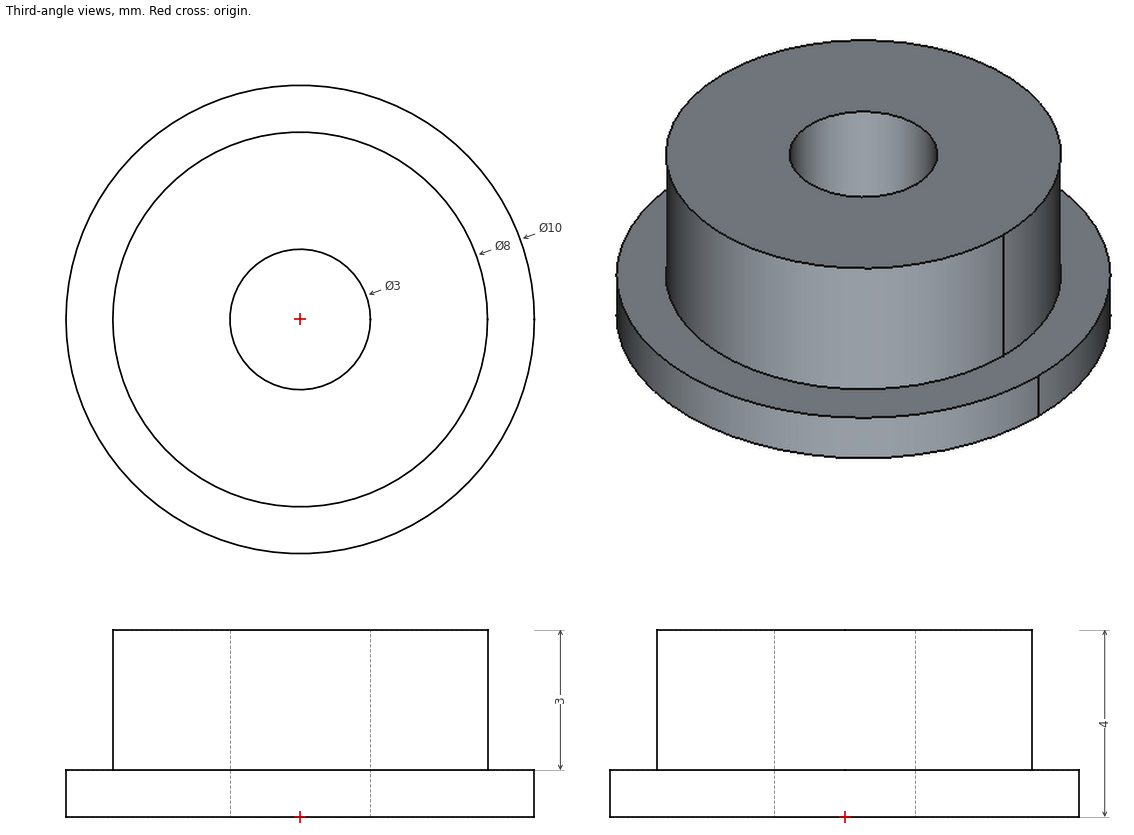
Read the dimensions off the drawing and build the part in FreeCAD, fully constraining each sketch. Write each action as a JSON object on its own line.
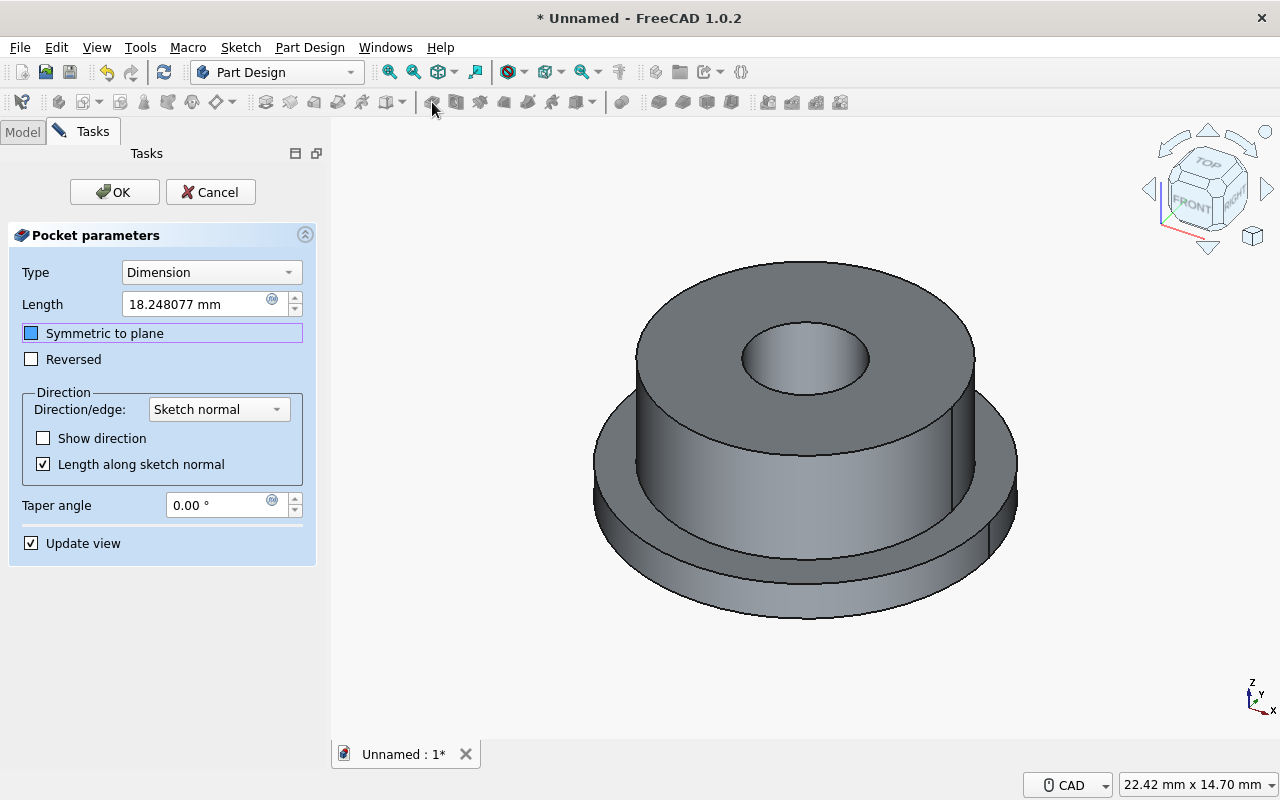
{"action": "left_click", "coordinate": [30, 333]}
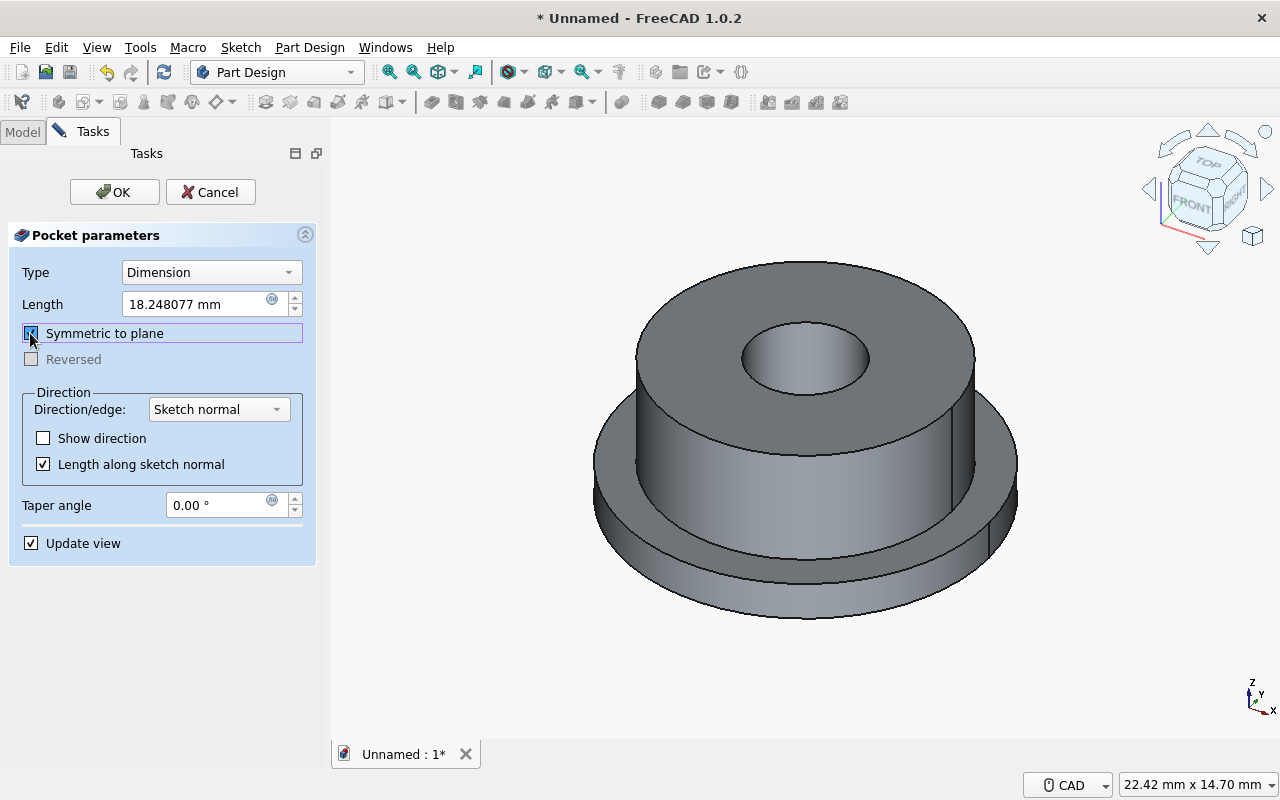
{"action": "left_click", "coordinate": [115, 192]}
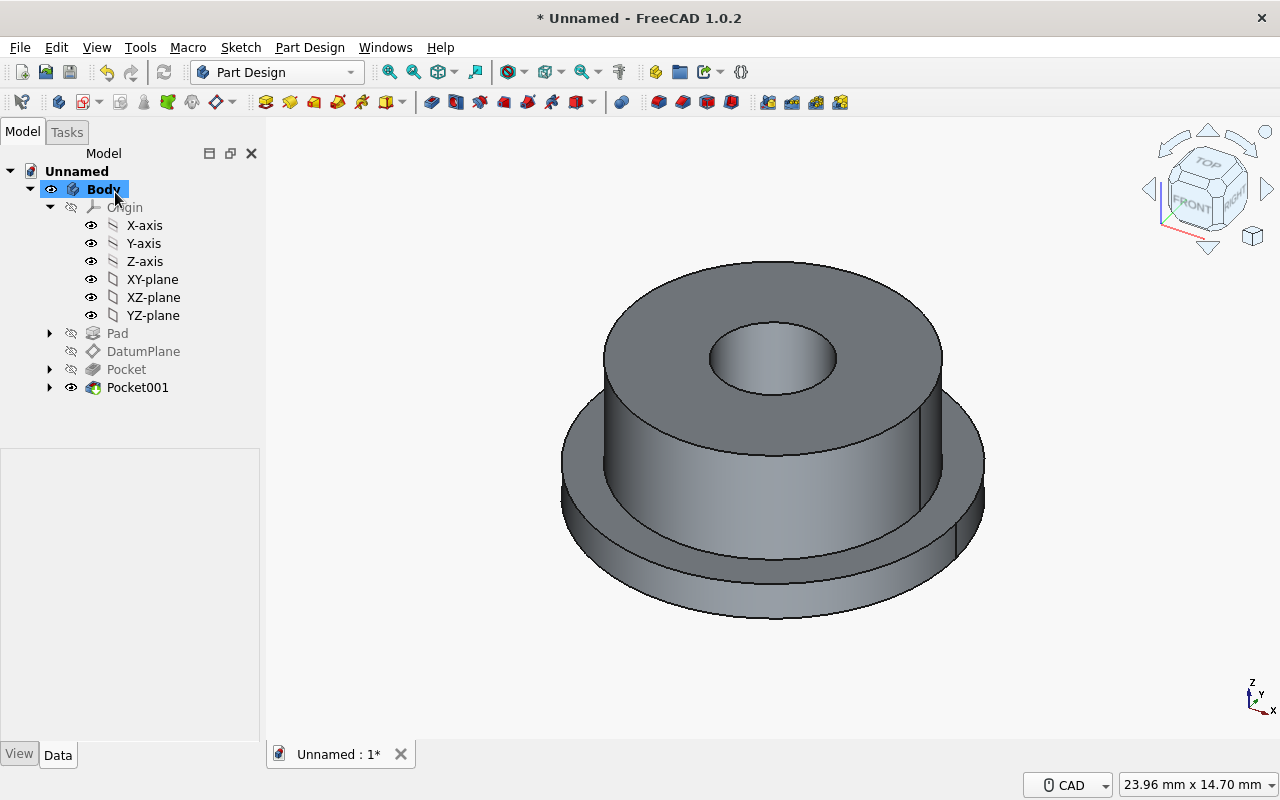
{"action": "key", "text": "0"}